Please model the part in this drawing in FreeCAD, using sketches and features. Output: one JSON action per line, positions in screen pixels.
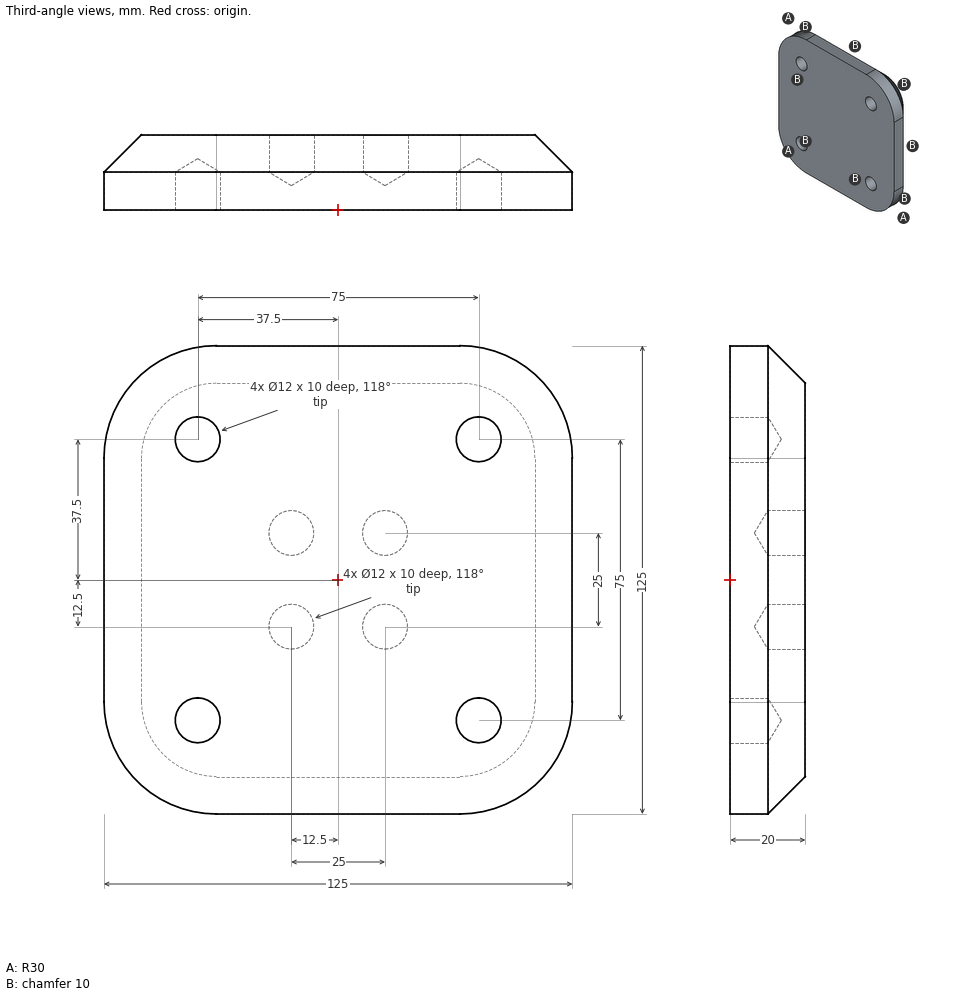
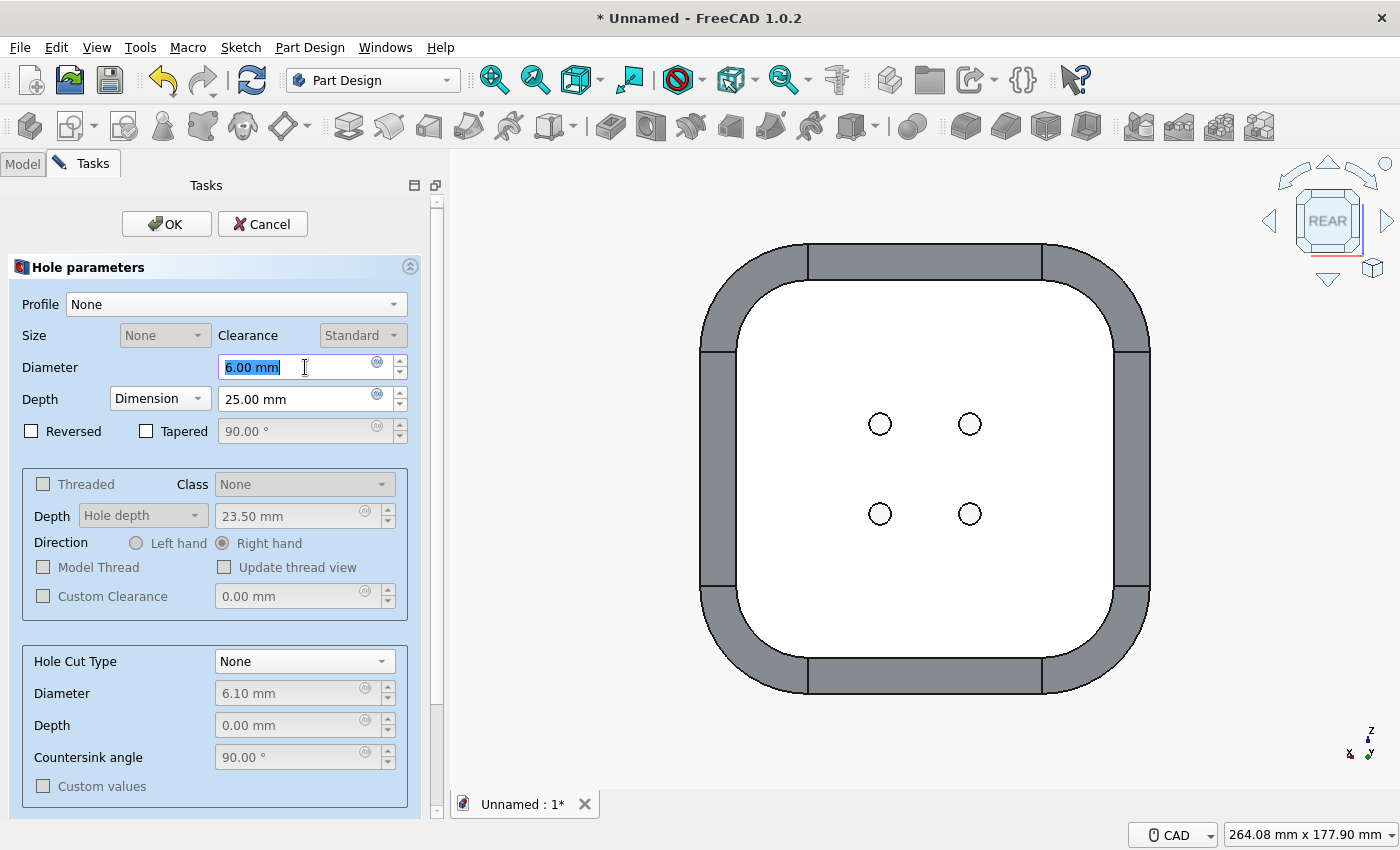
{"action": "type", "text": "12"}
{"action": "key", "text": "Tab"}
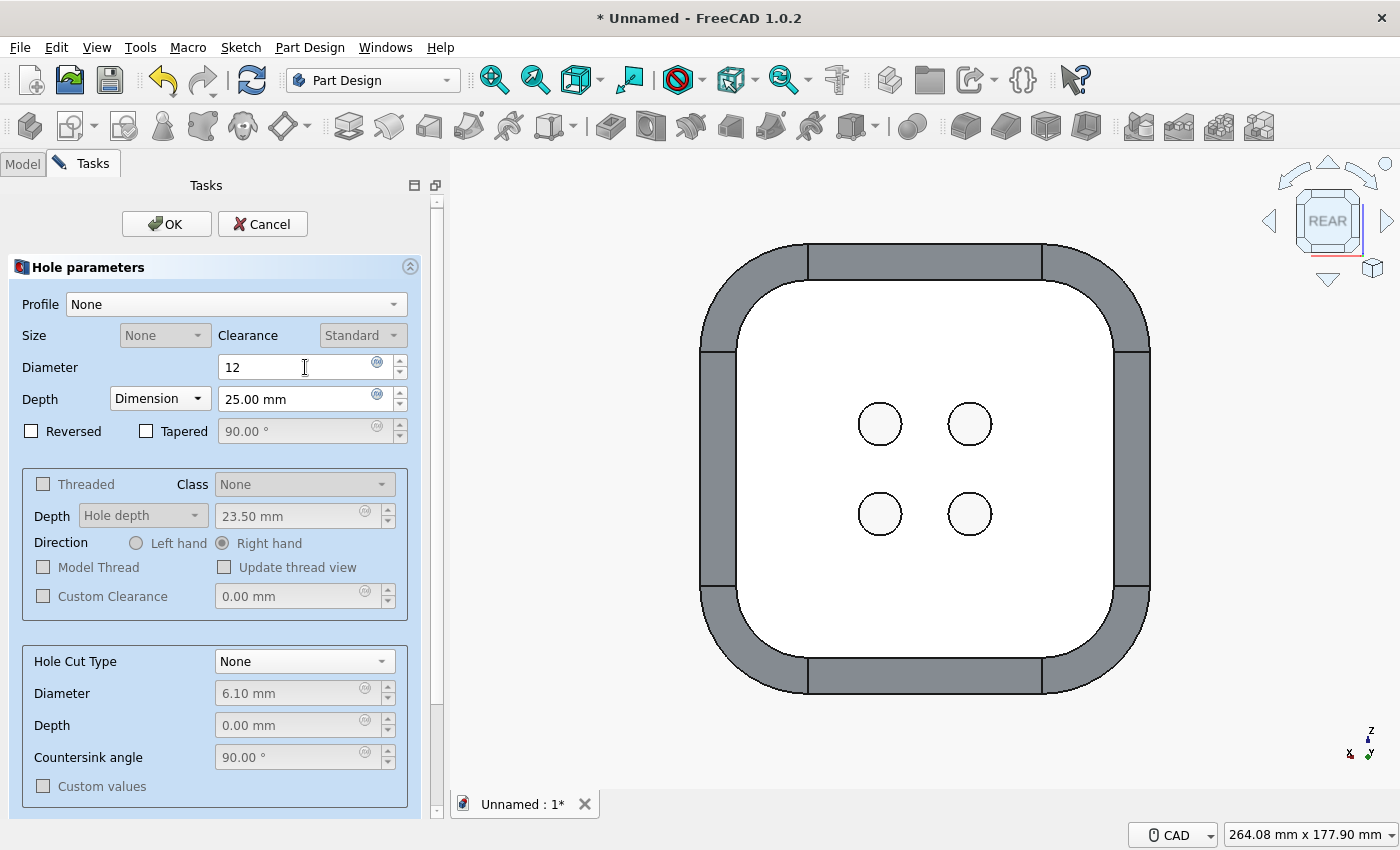
{"action": "triple_click", "coordinate": [305, 399]}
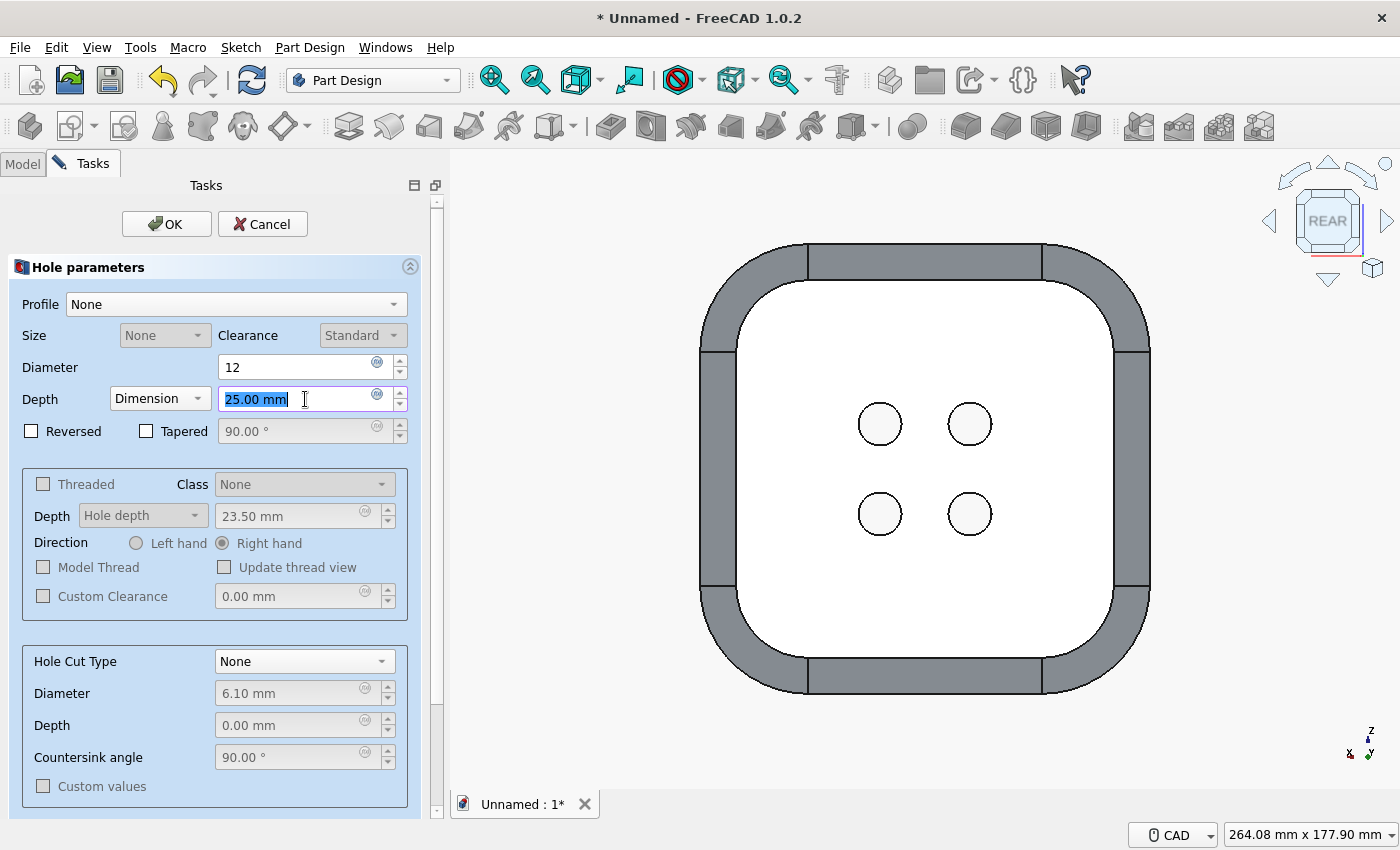
{"action": "type", "text": "10"}
{"action": "key", "text": "Tab"}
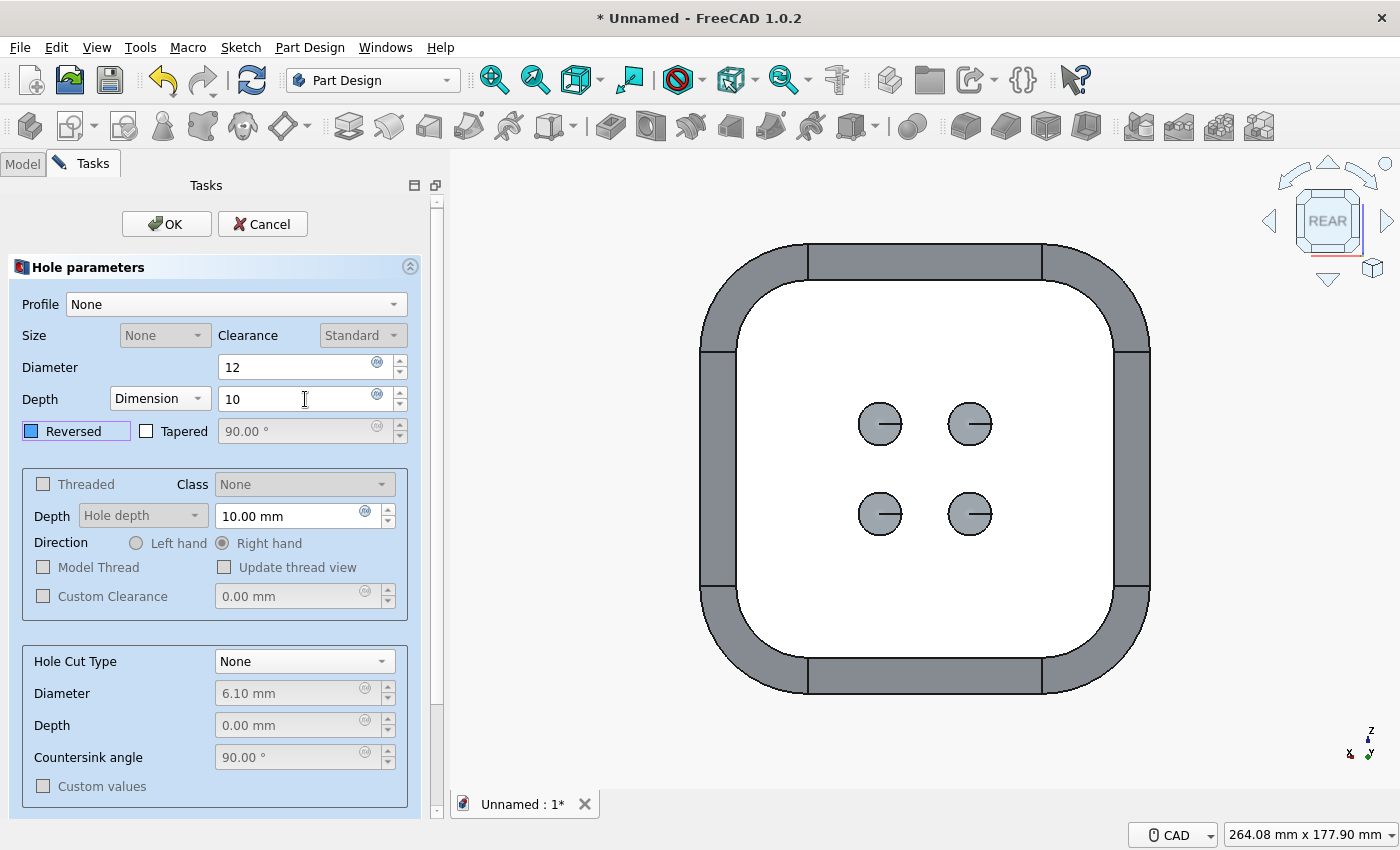
{"action": "left_click", "coordinate": [167, 224]}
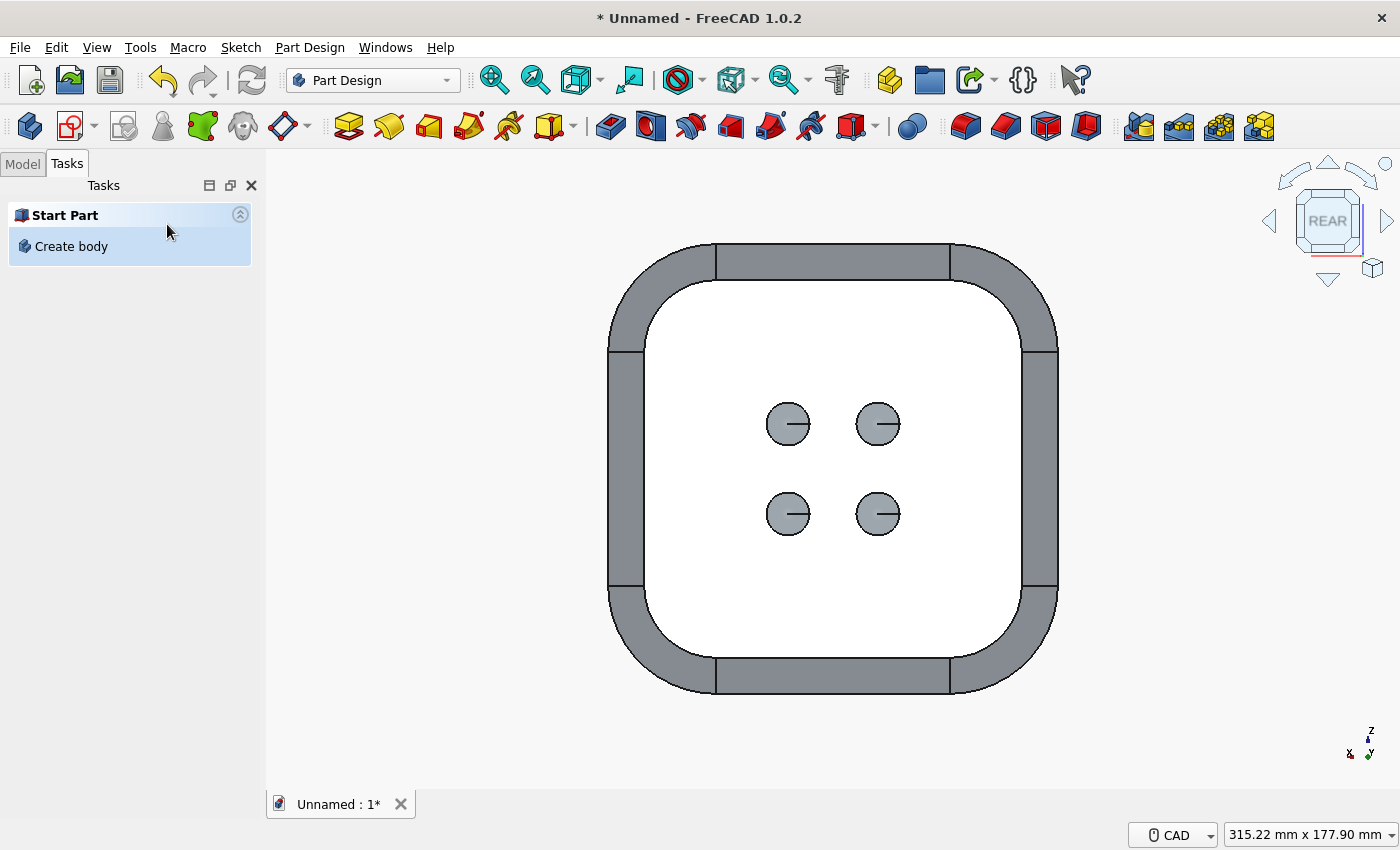
{"action": "left_click", "coordinate": [70, 126]}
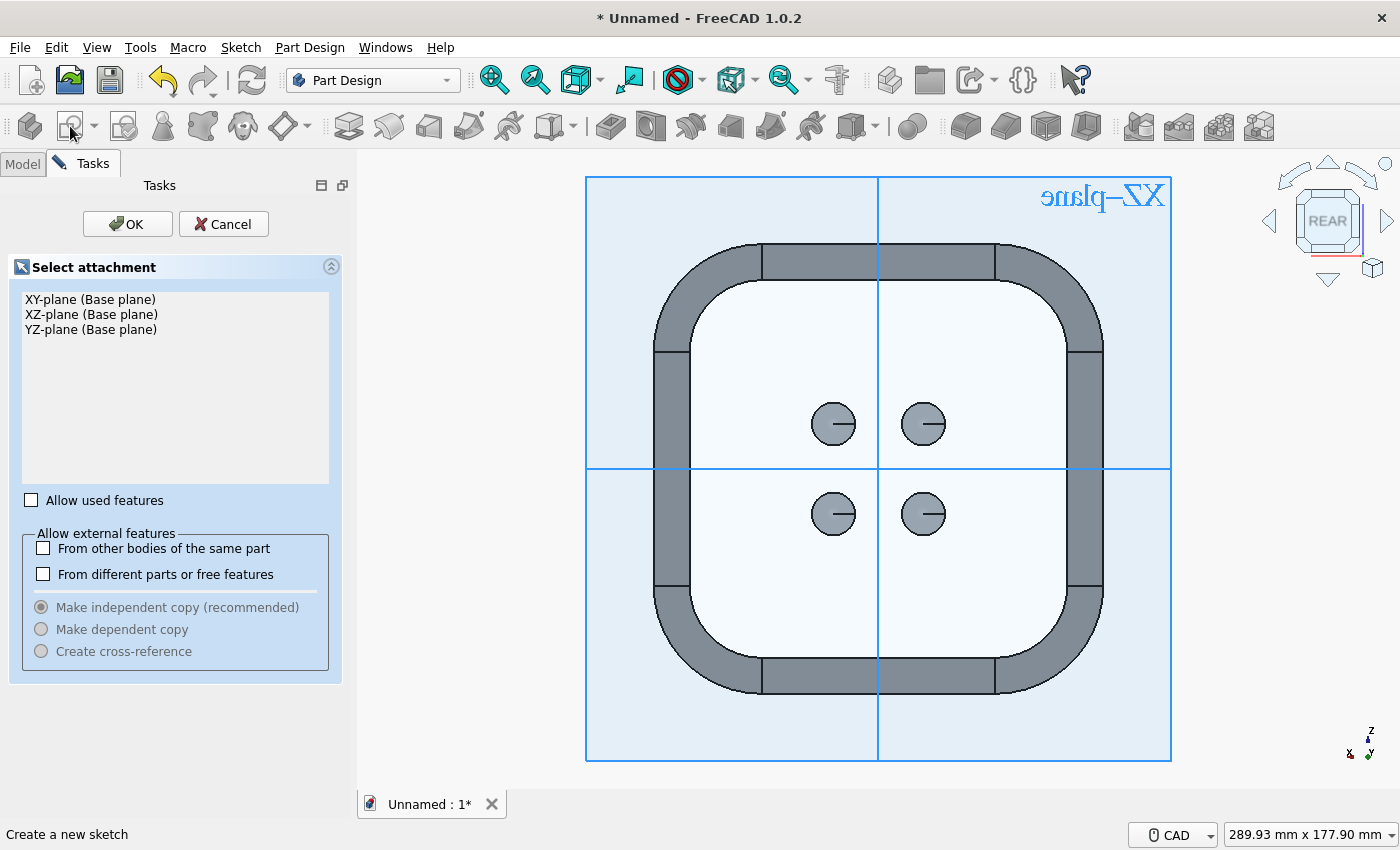
{"action": "left_click", "coordinate": [82, 314]}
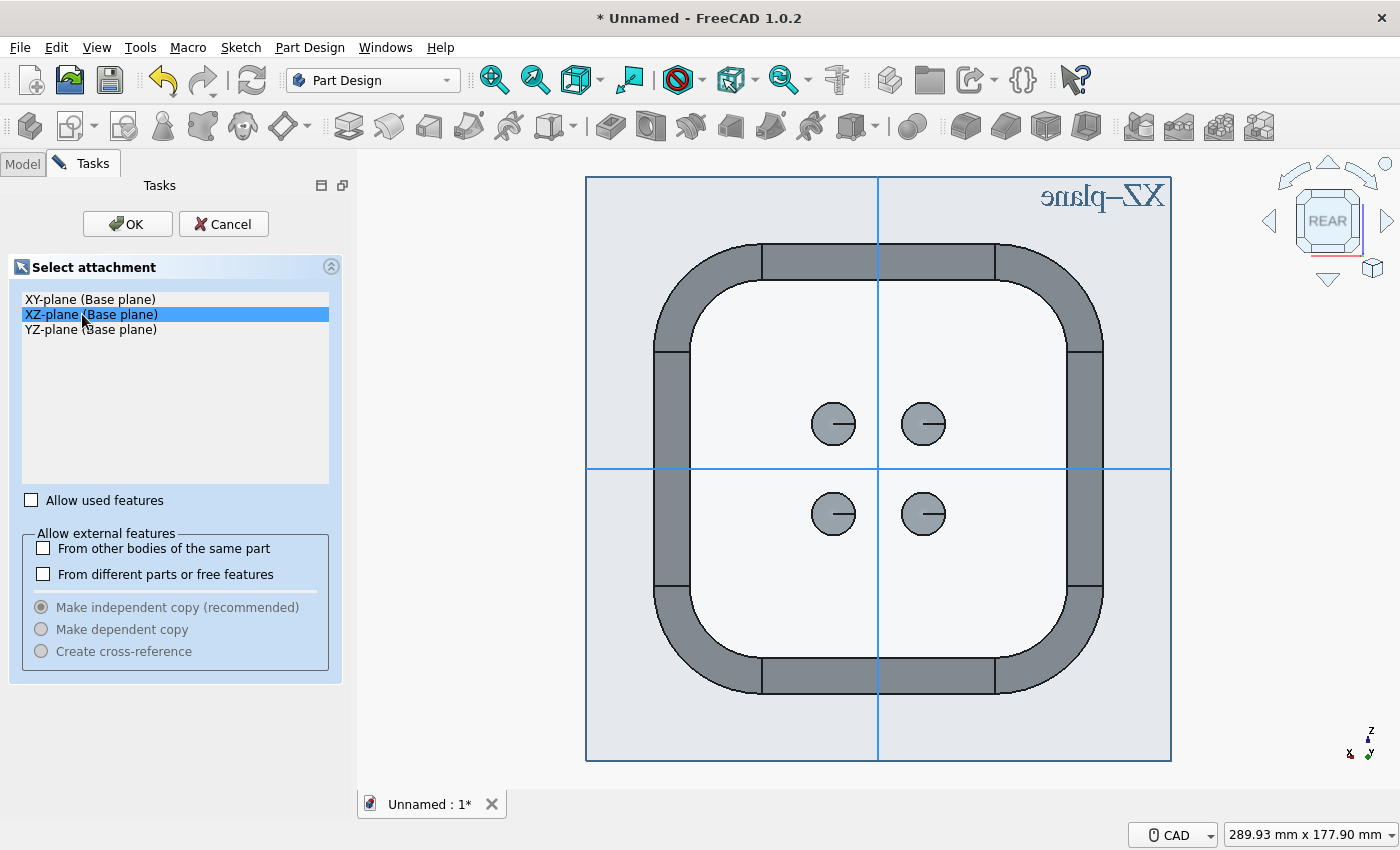
{"action": "left_click", "coordinate": [128, 224]}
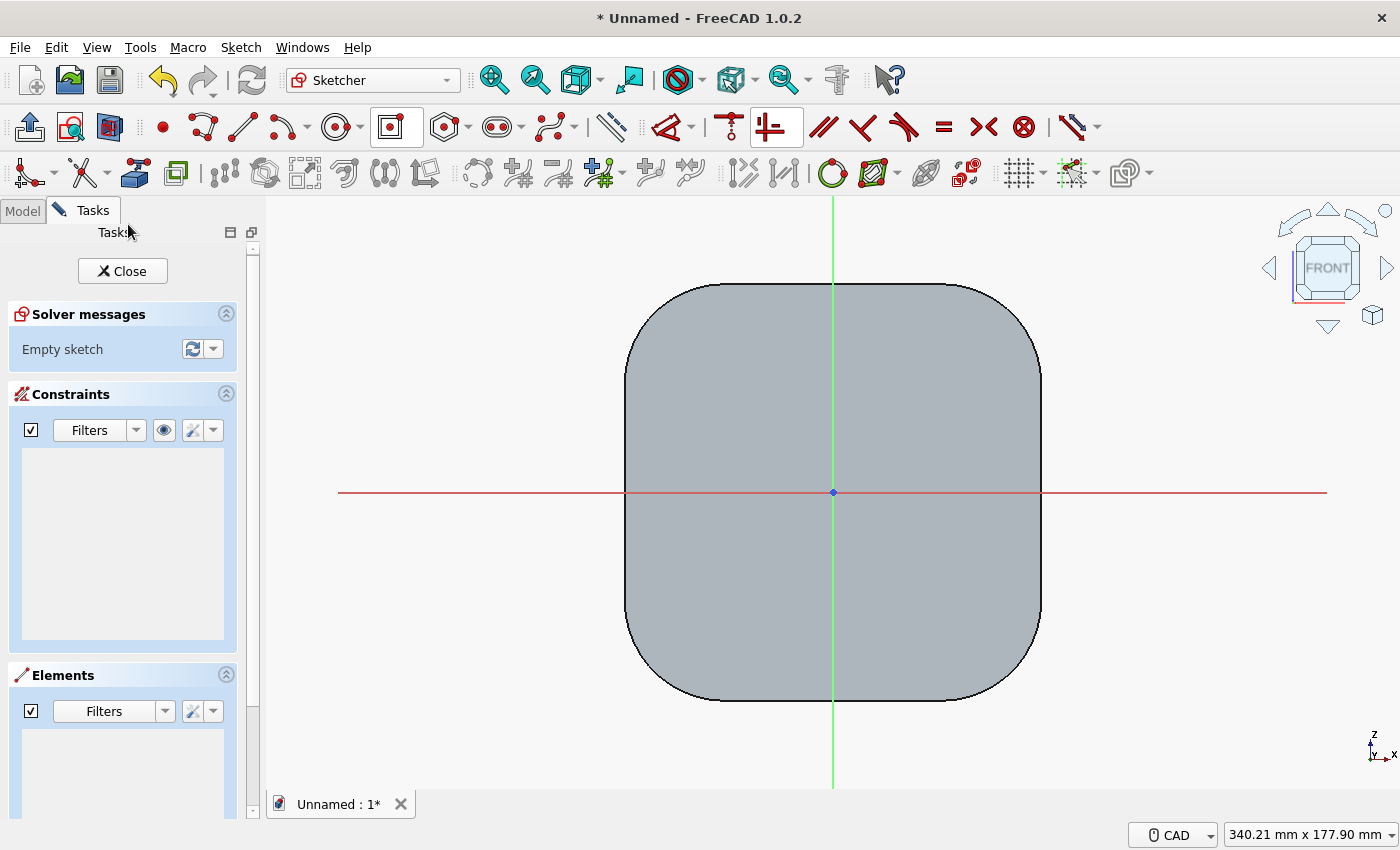
{"action": "key", "text": "g c"}